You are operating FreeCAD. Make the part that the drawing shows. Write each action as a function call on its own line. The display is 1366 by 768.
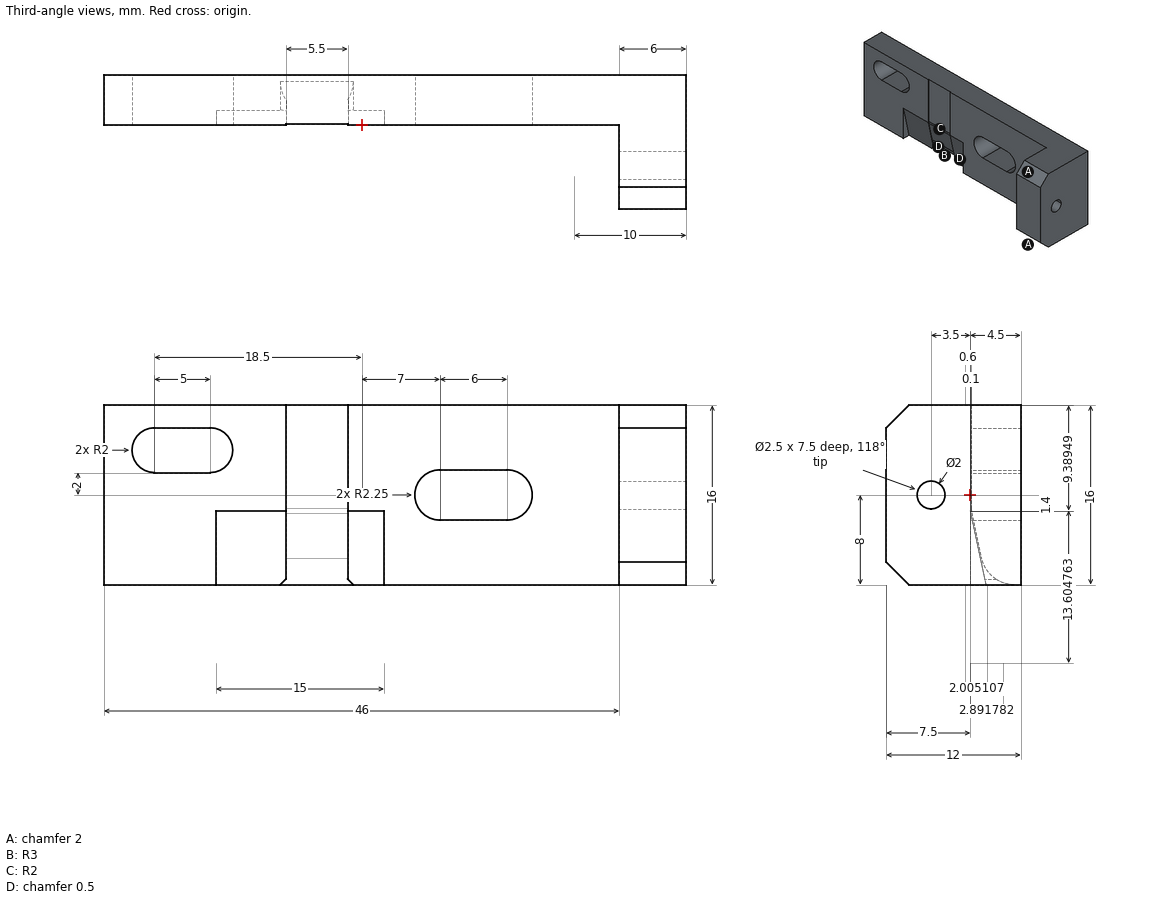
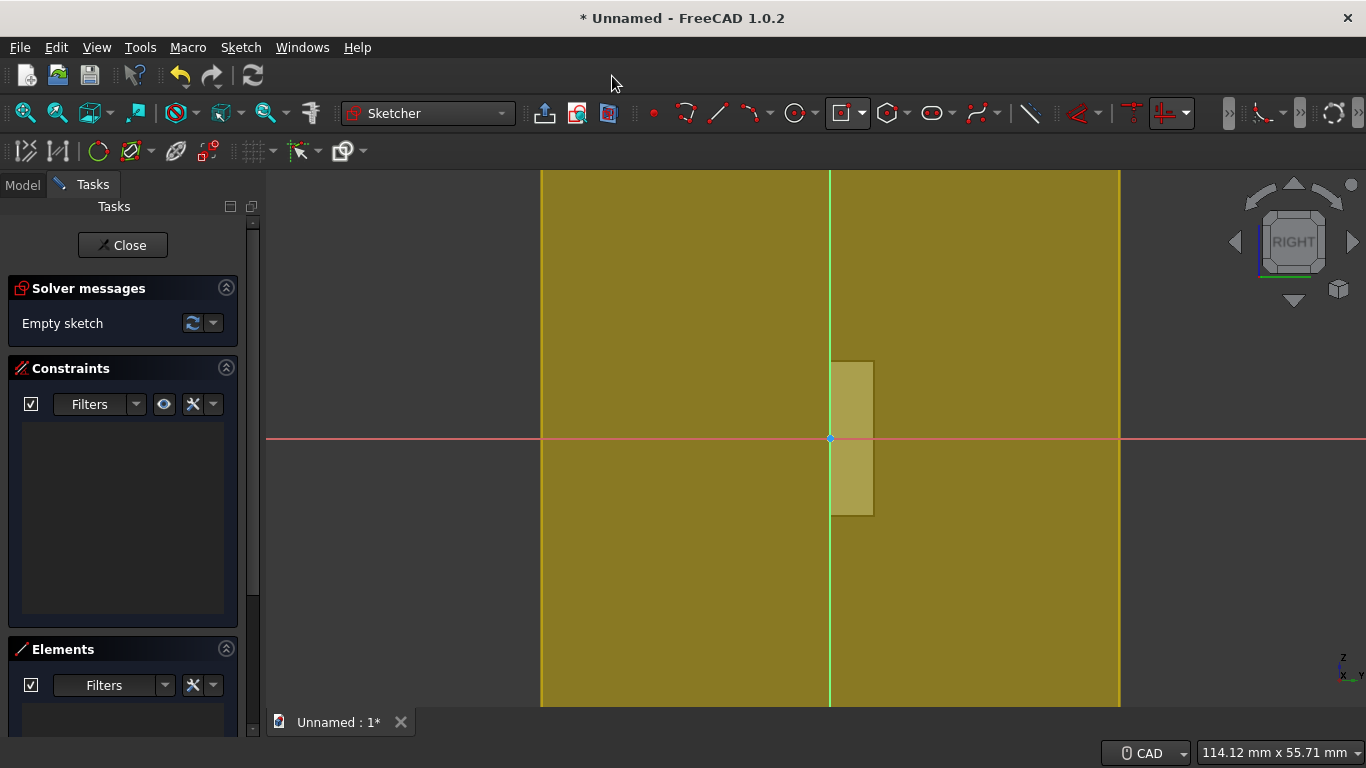
scroll(923, 570, up, 4)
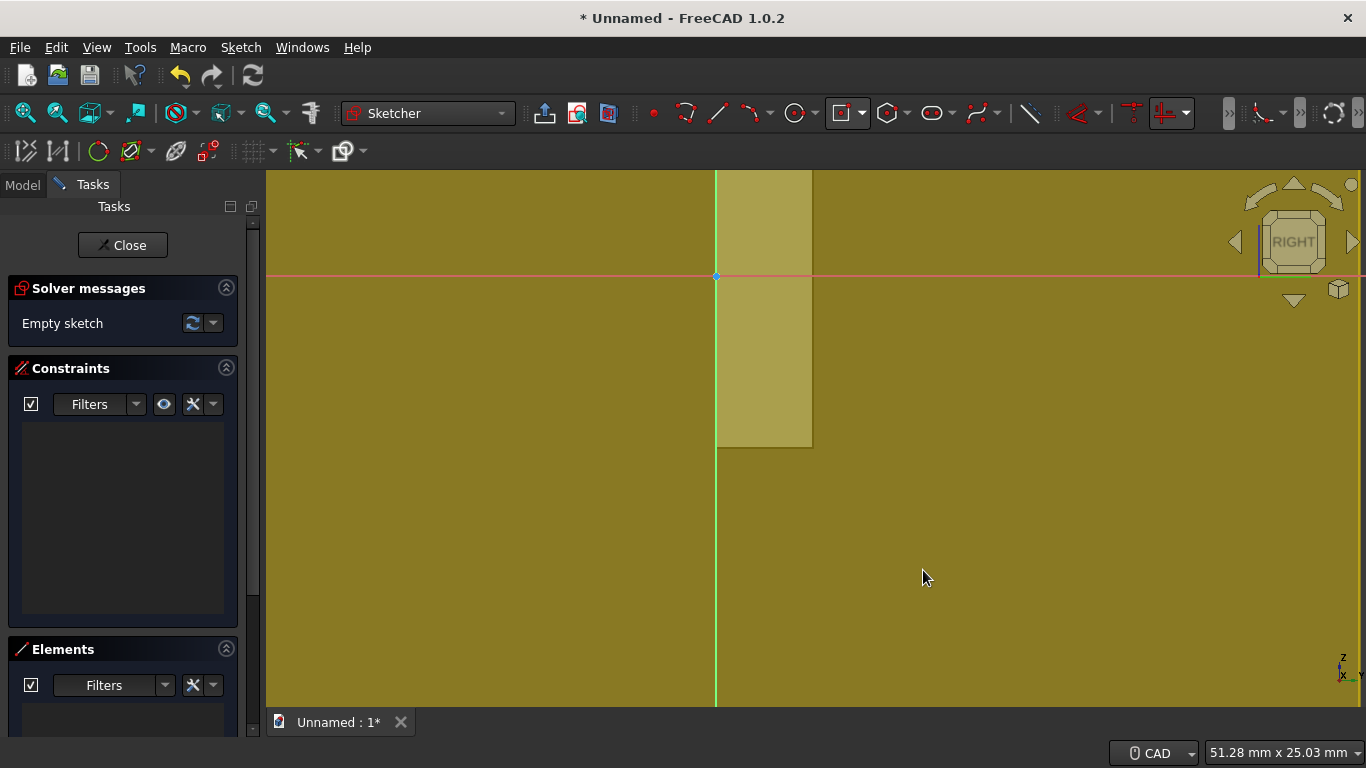
click(686, 114)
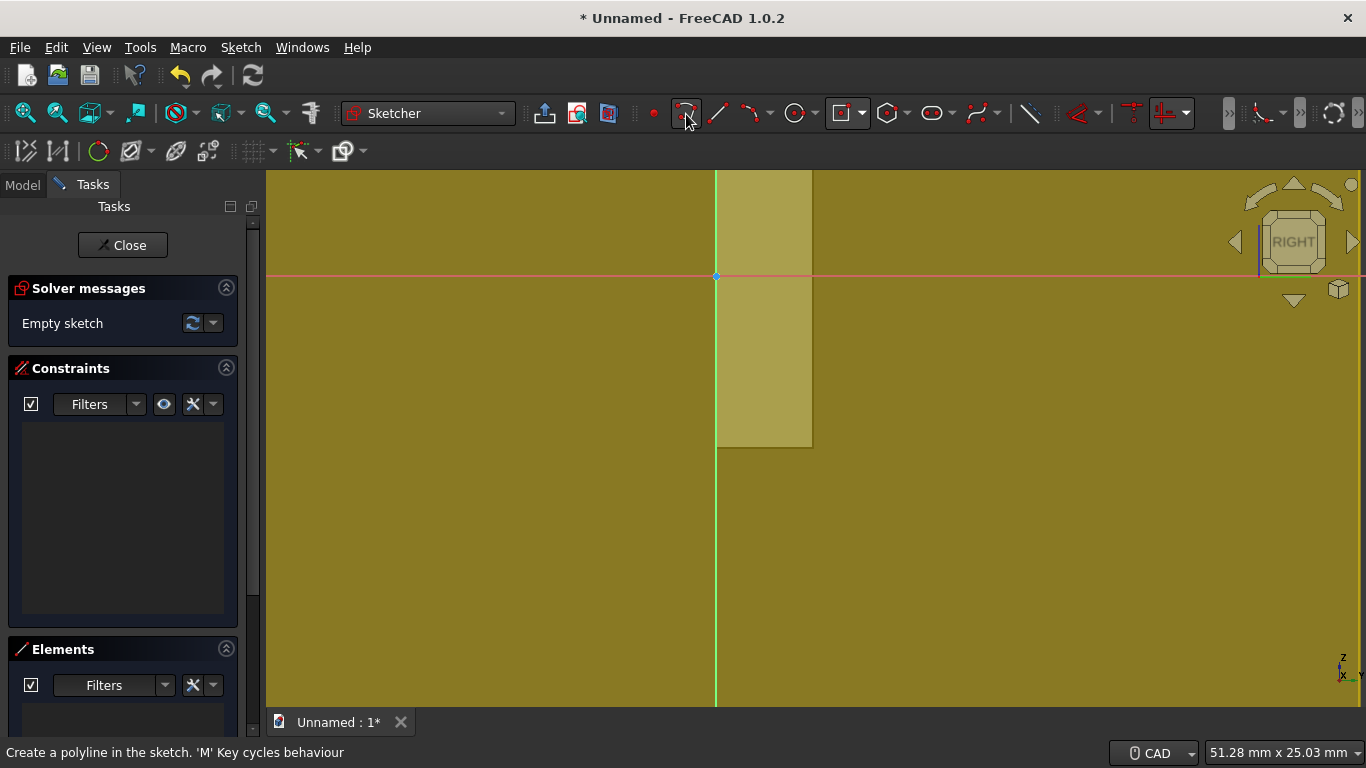
click(716, 306)
click(778, 598)
click(725, 598)
click(716, 307)
key(Escape)
key(Escape)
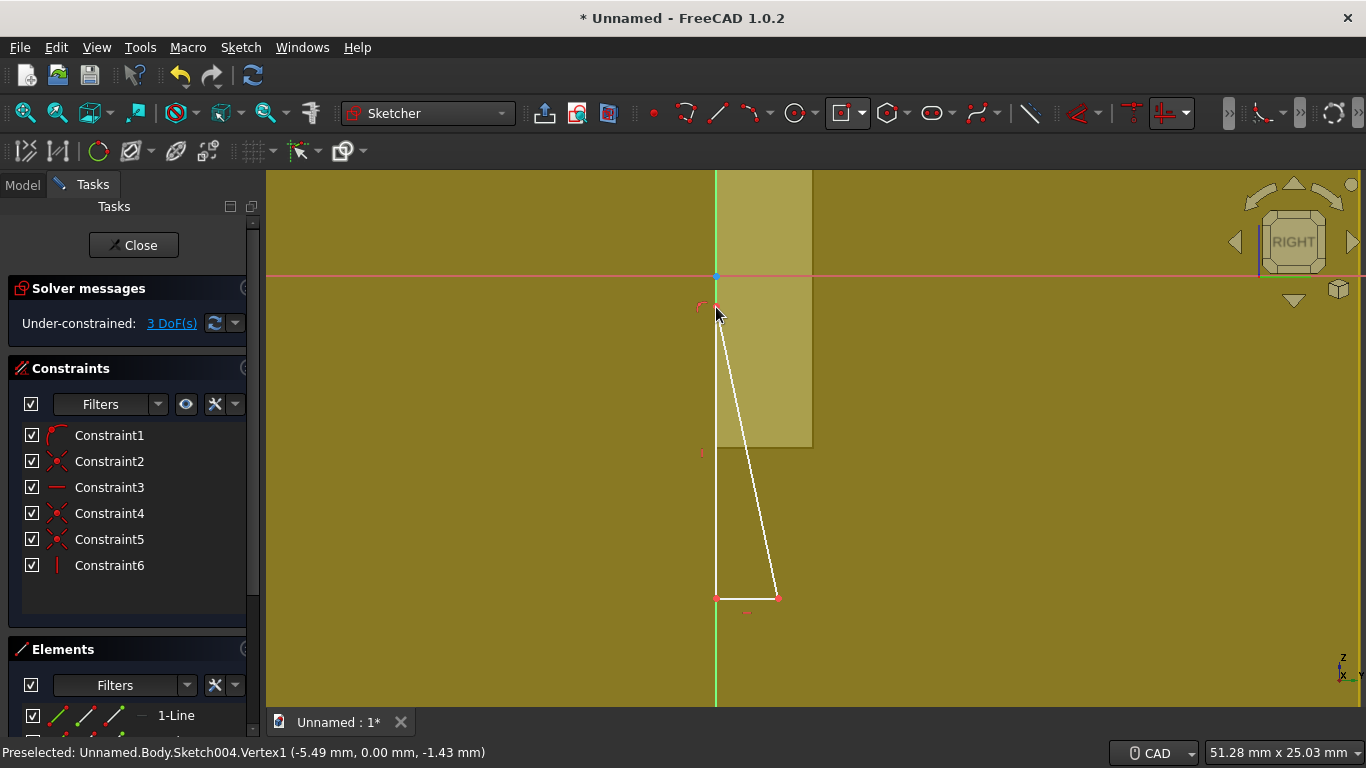
key(d)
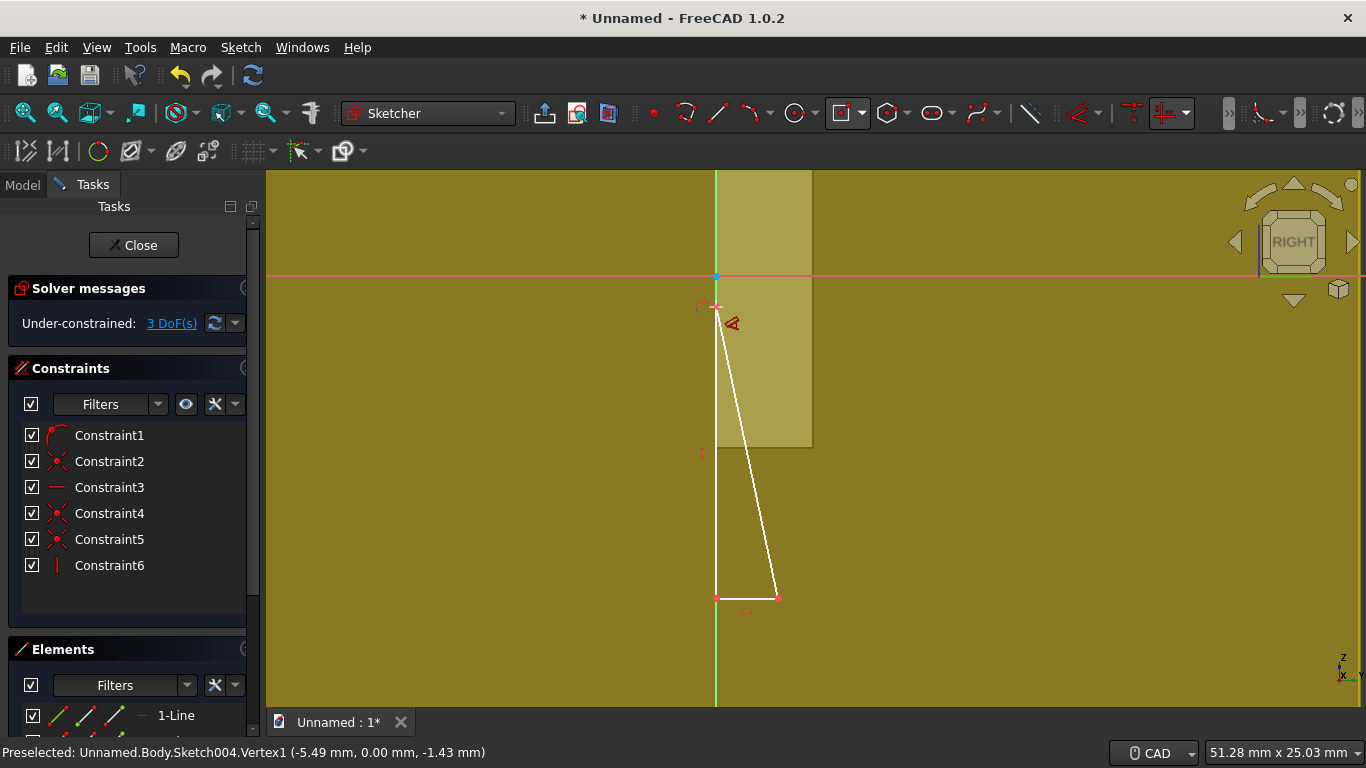
scroll(716, 307, up, 2)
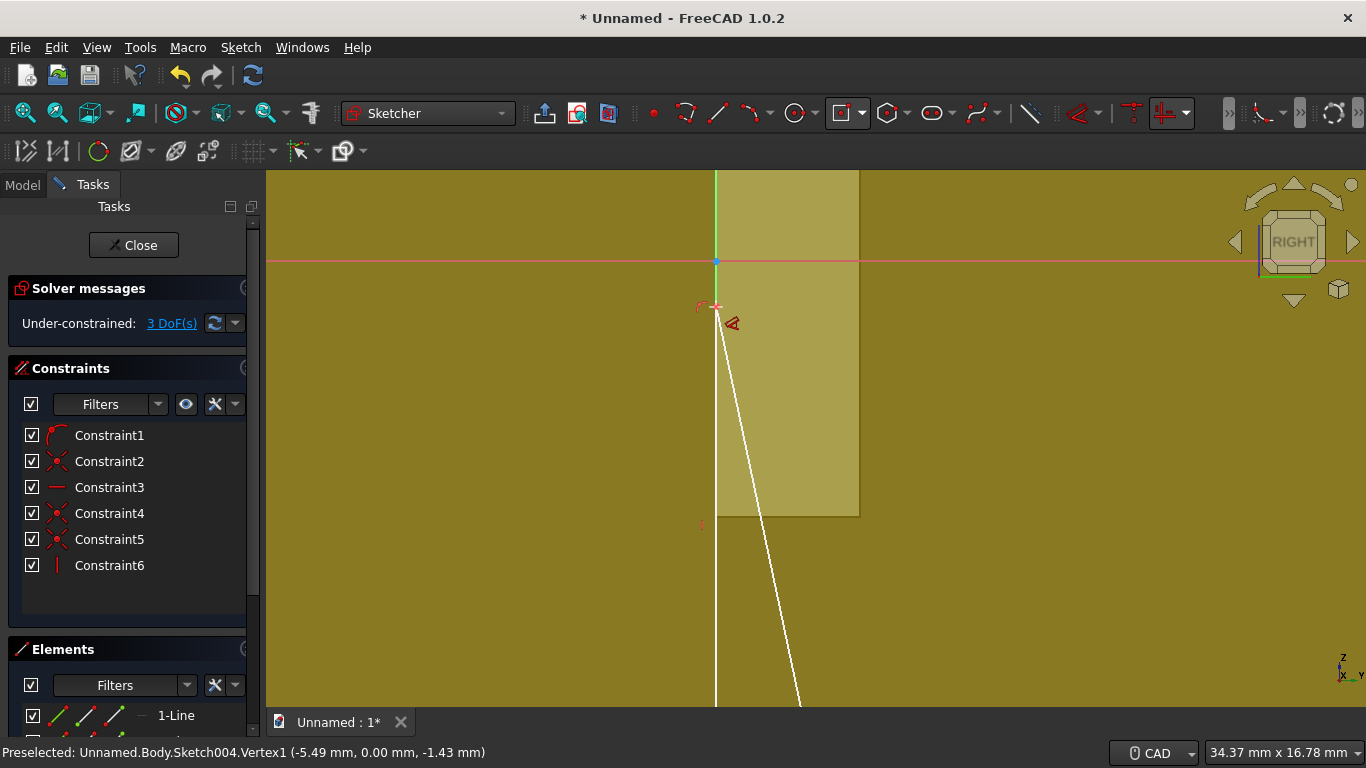
click(716, 307)
click(682, 284)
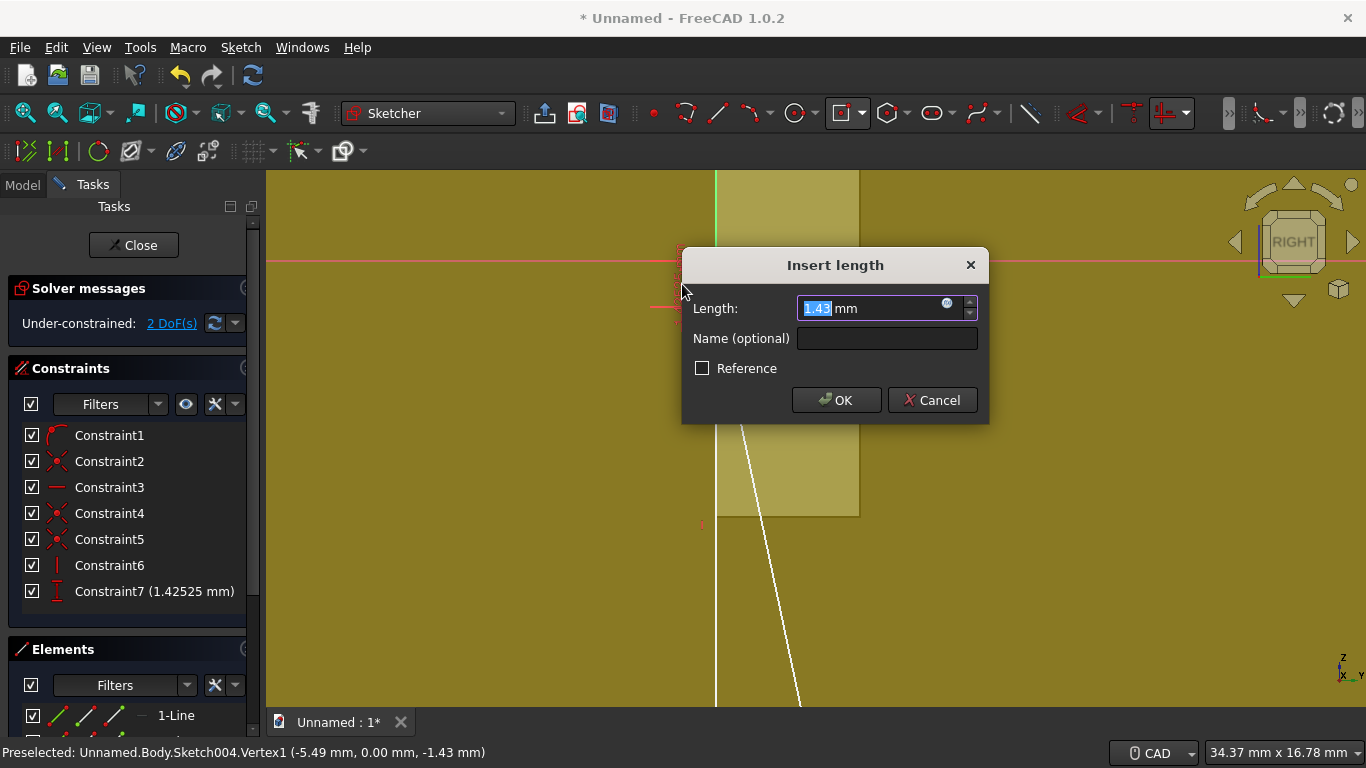
text(1.4)
key(Return)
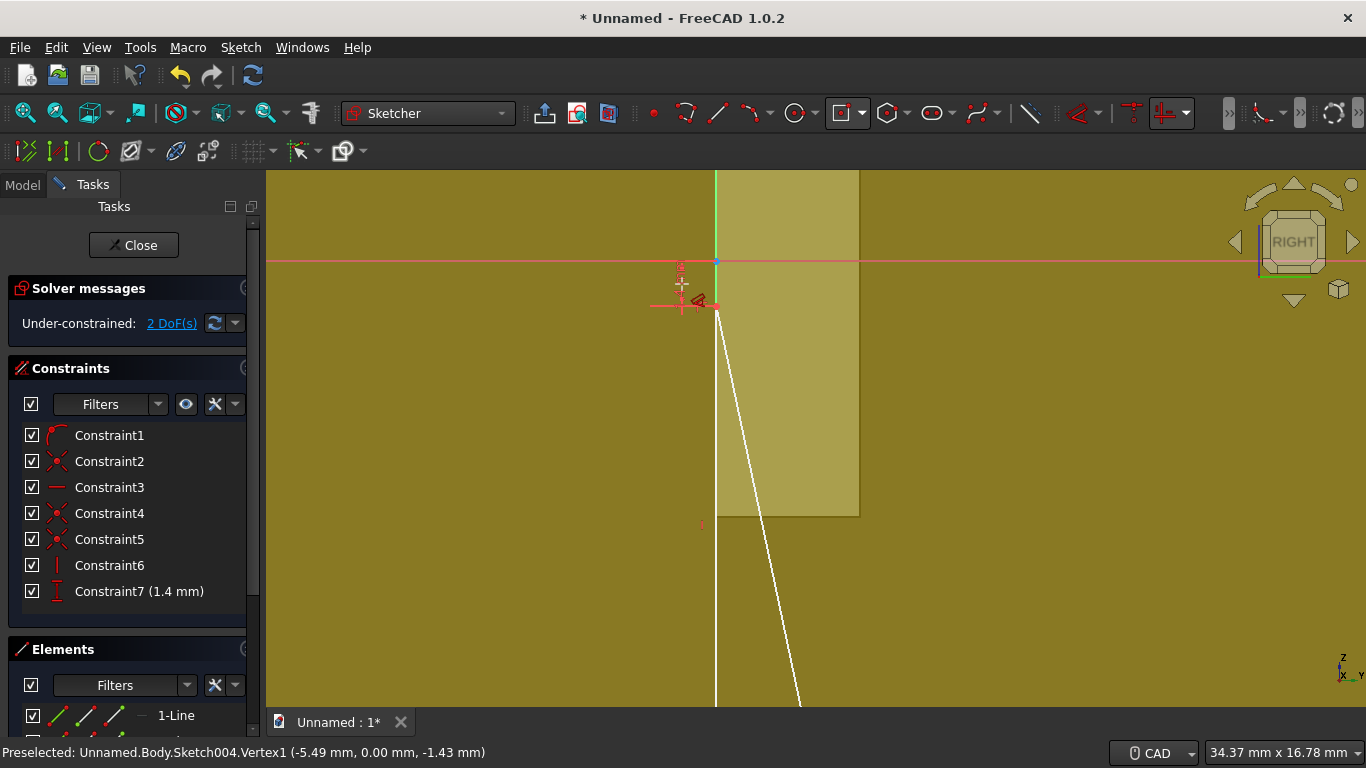
scroll(717, 311, down, 2)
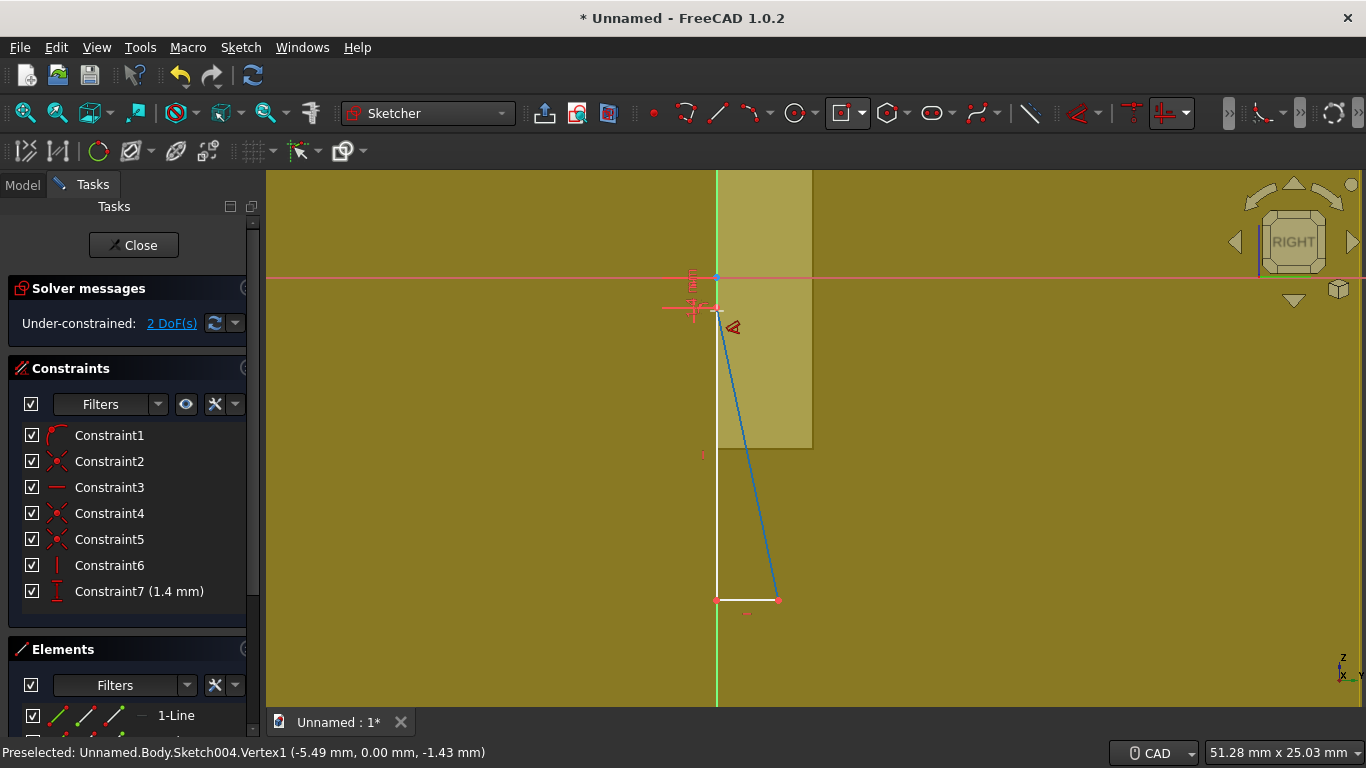
click(760, 600)
click(747, 634)